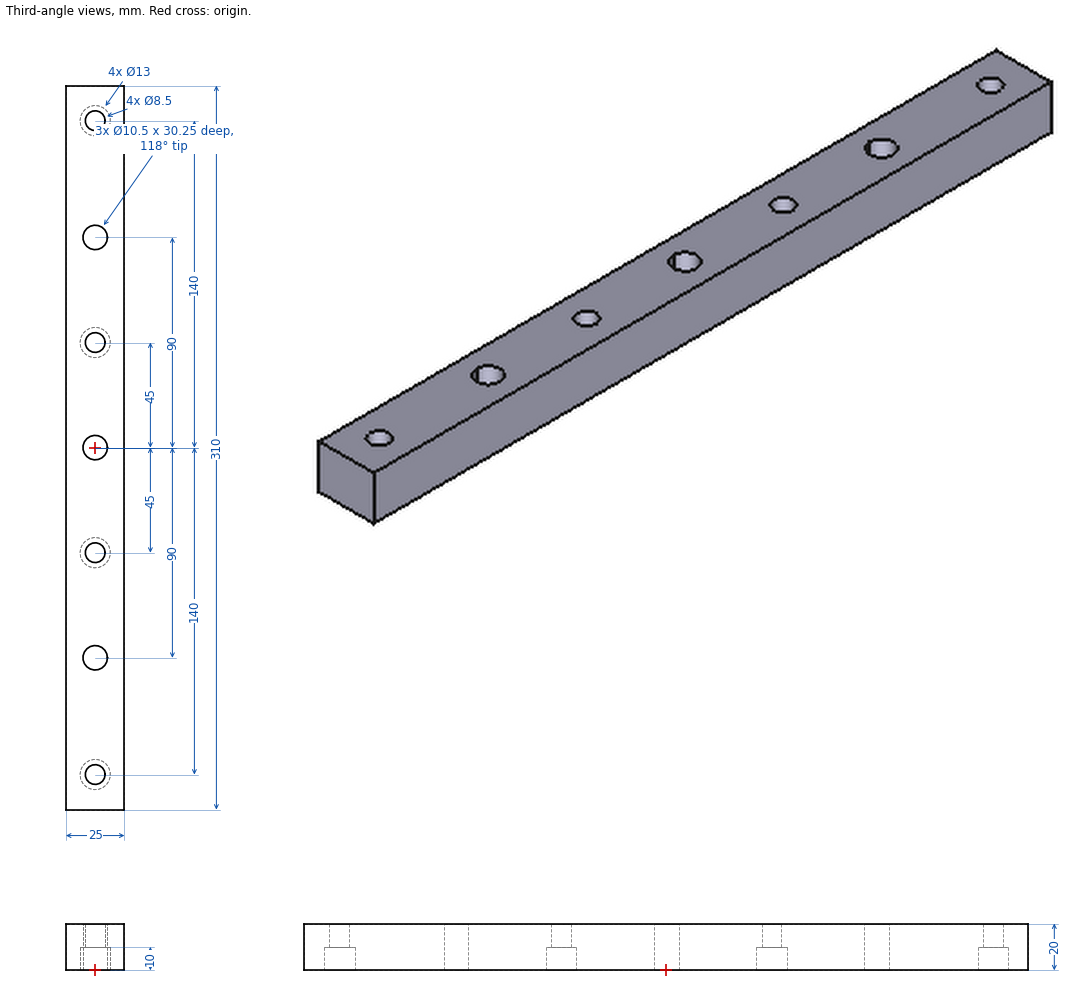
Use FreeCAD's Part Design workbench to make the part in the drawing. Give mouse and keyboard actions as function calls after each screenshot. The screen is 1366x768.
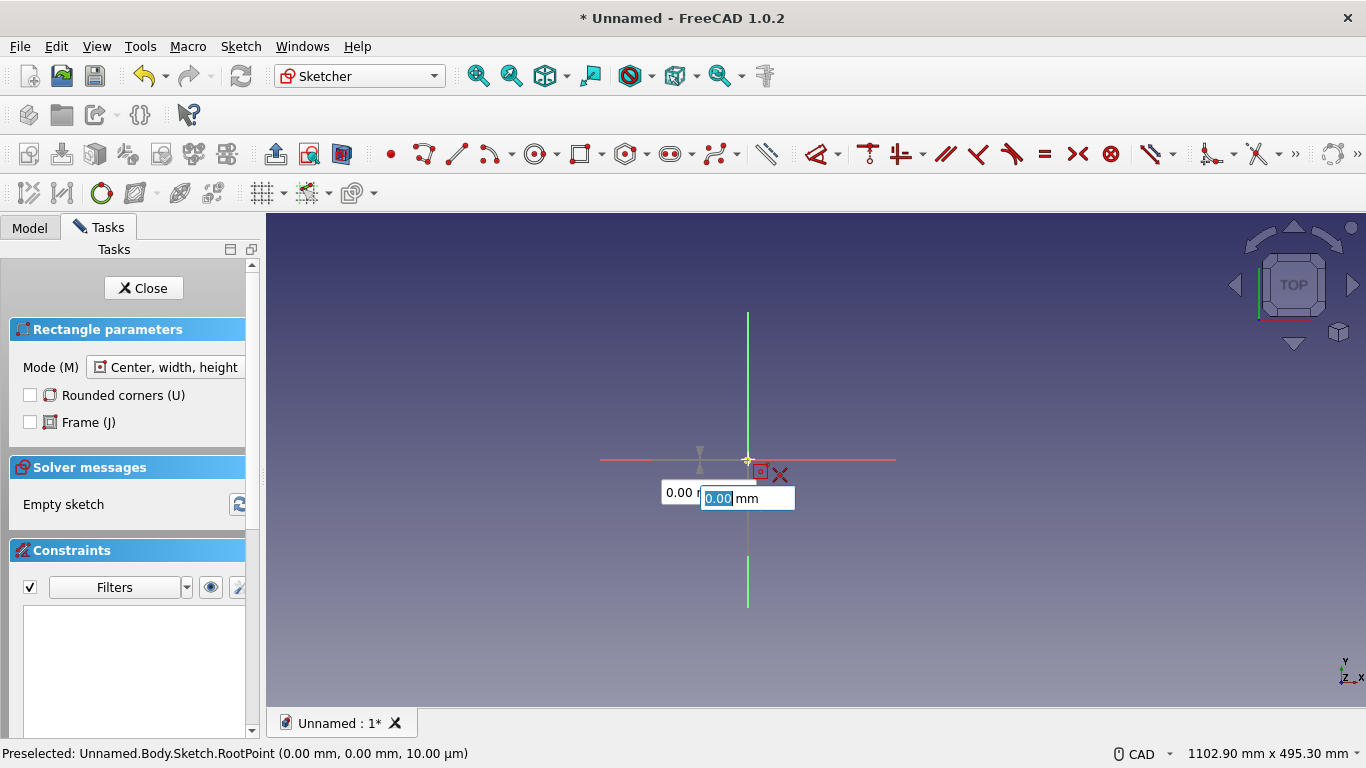
scroll(760, 305, up, 2)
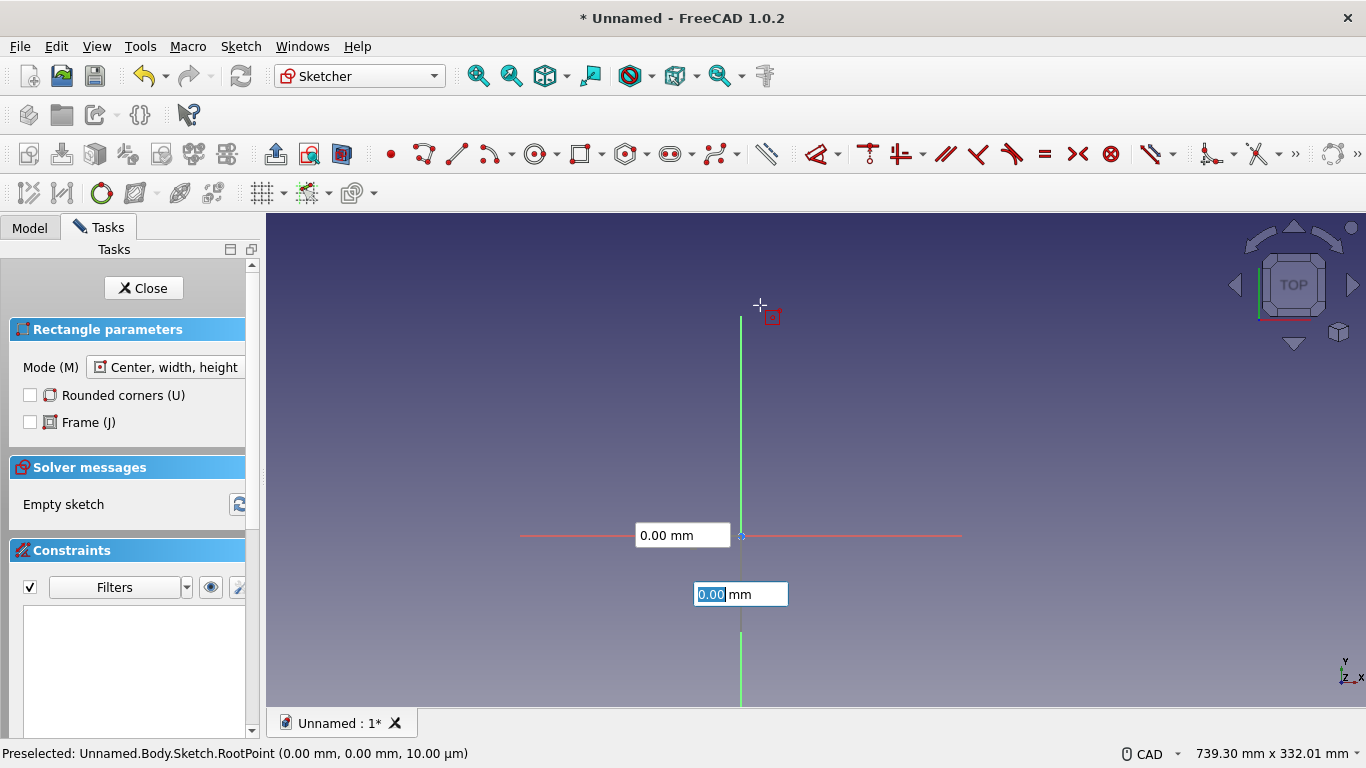
click(760, 306)
key(Escape)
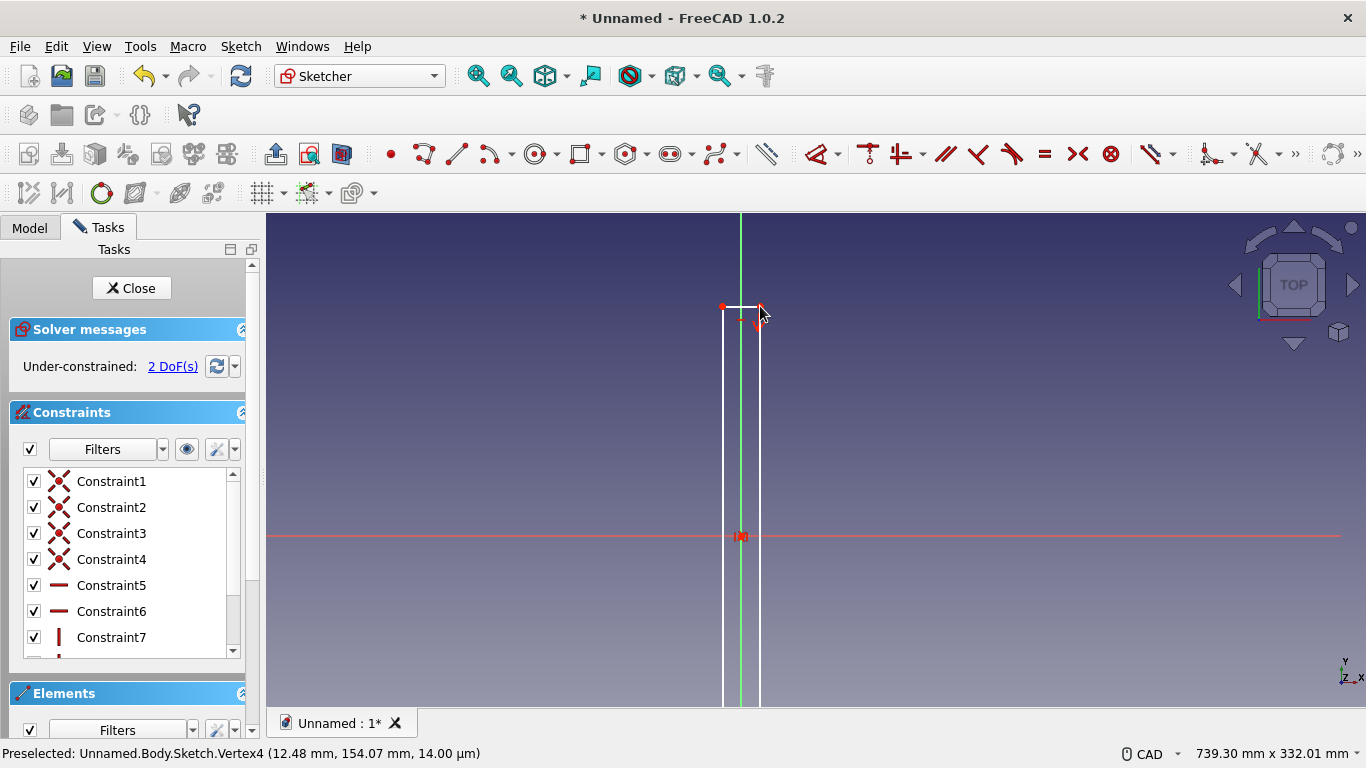
key(d)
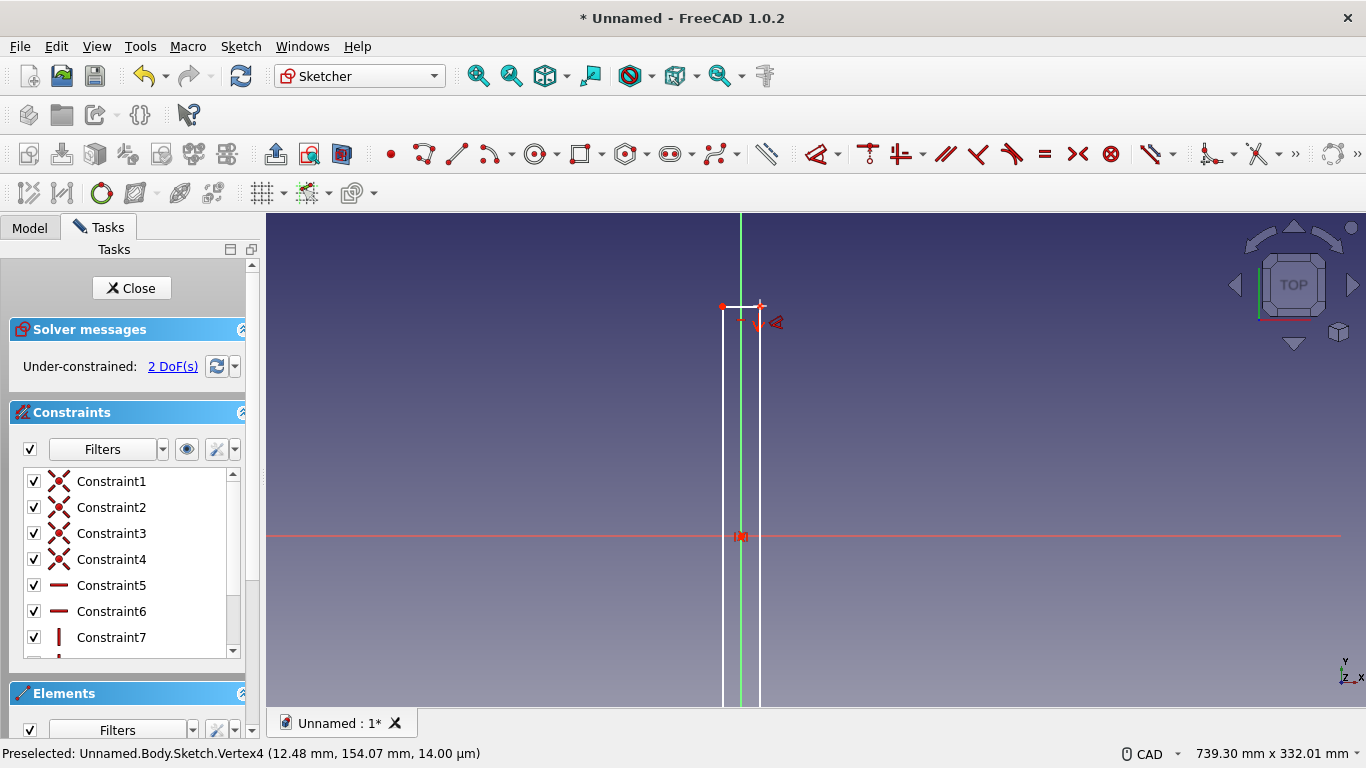
scroll(760, 305, down, 2)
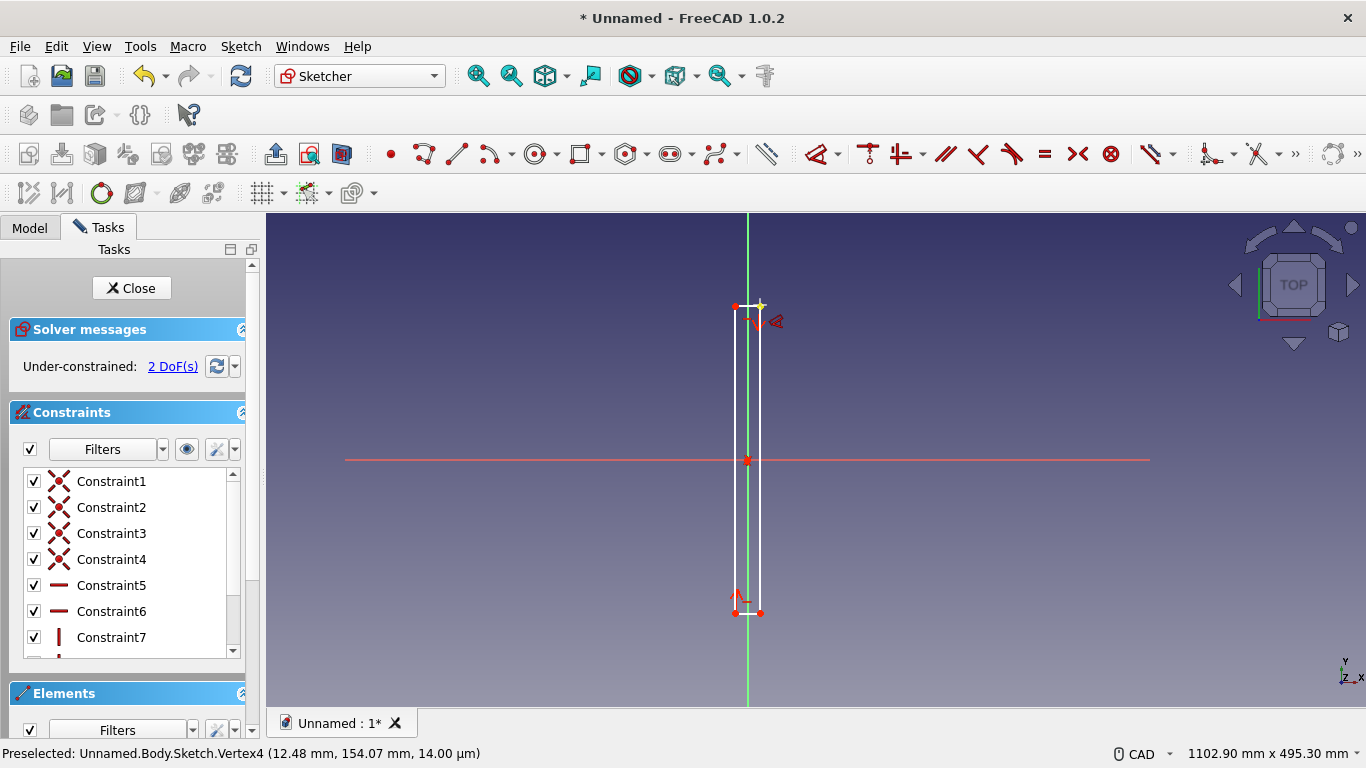
scroll(745, 614, up, 3)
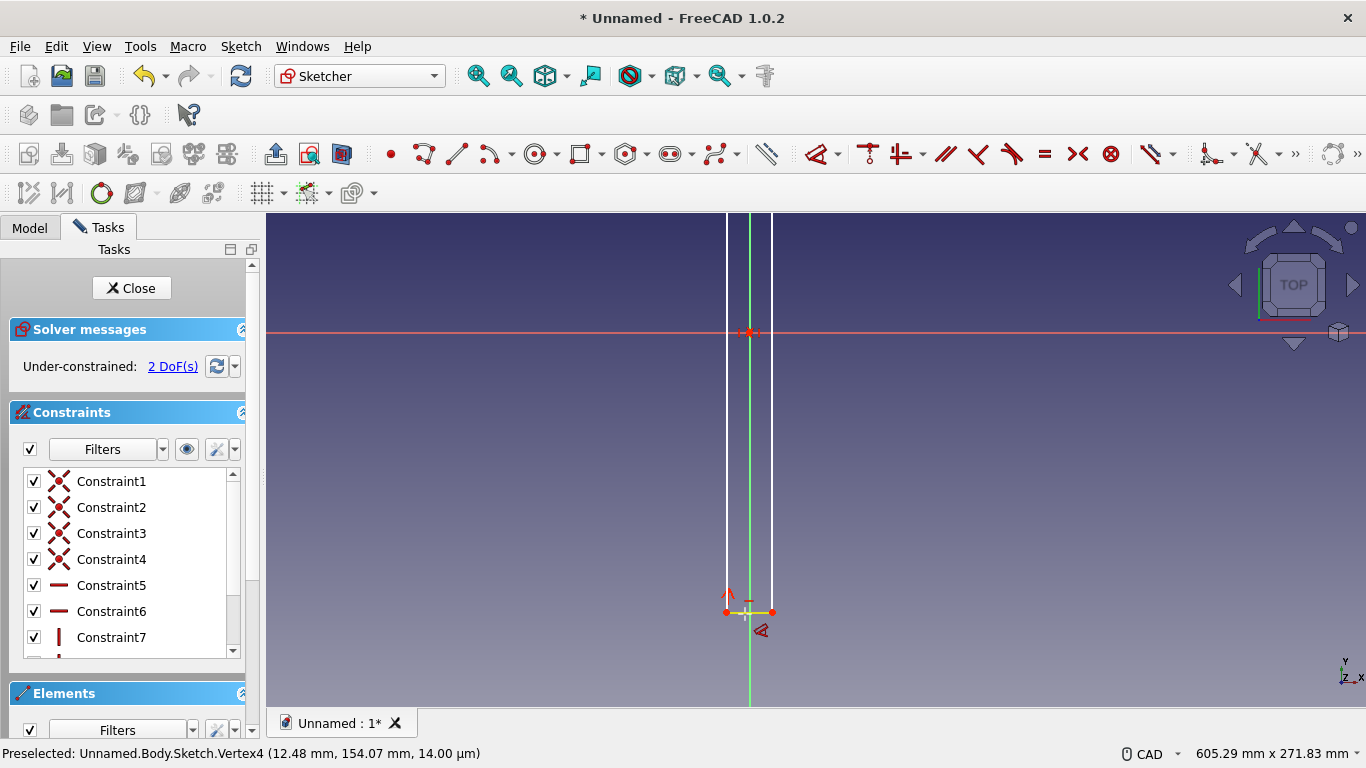
click(745, 613)
click(734, 647)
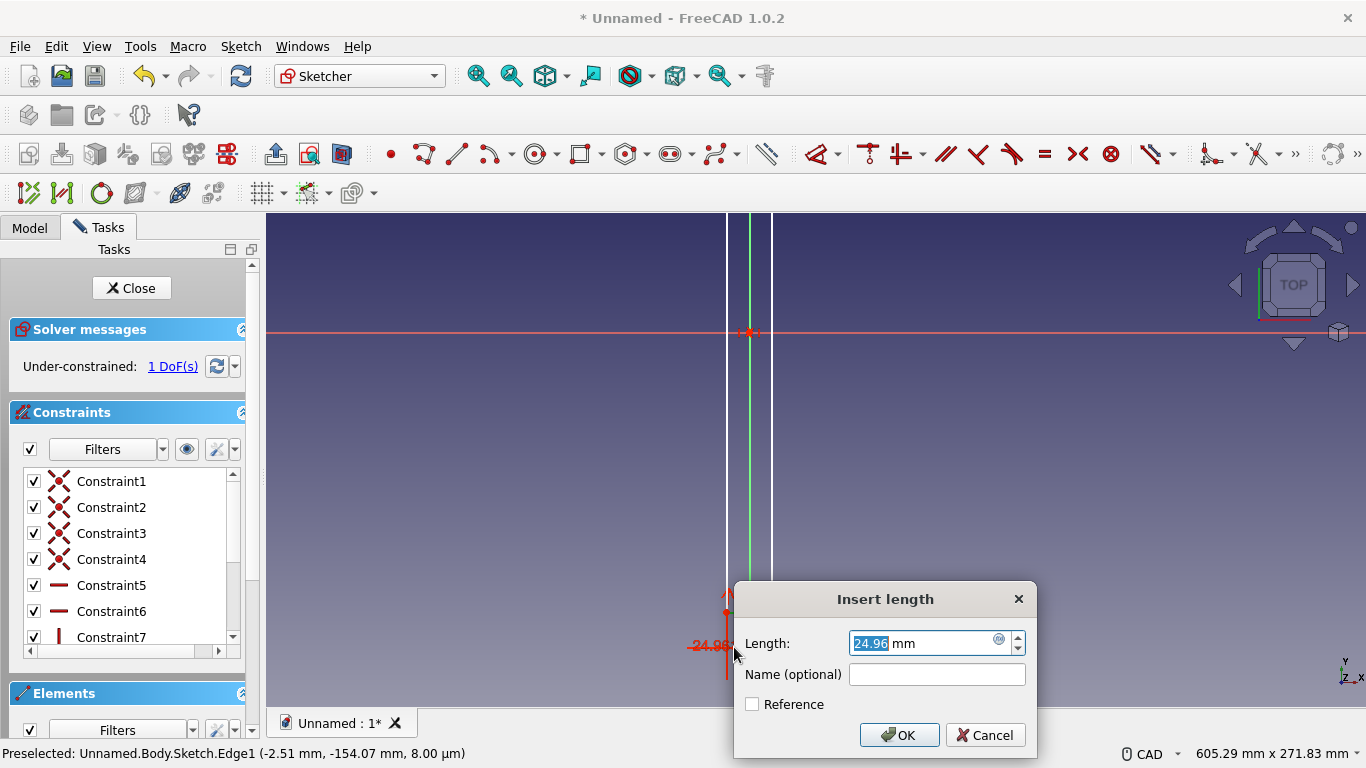
text(25)
key(Return)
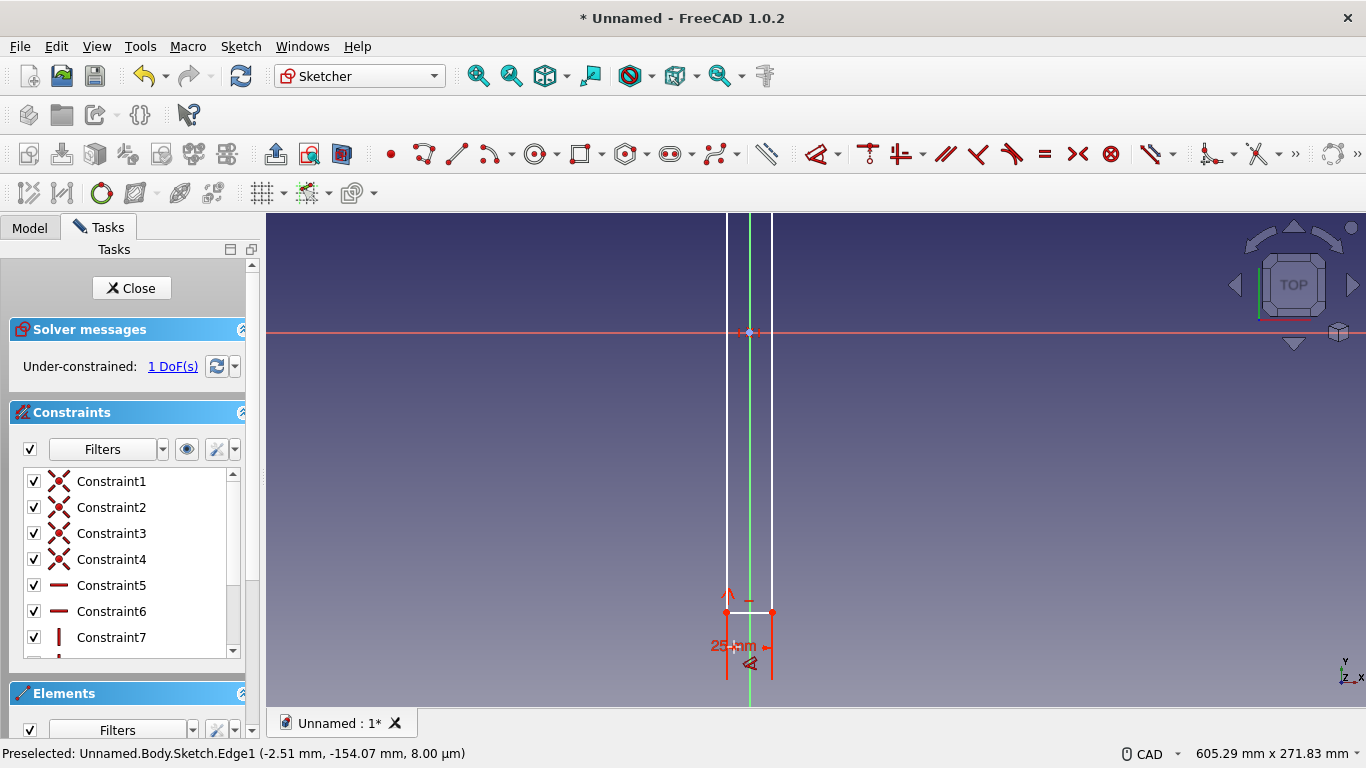
click(772, 445)
click(806, 427)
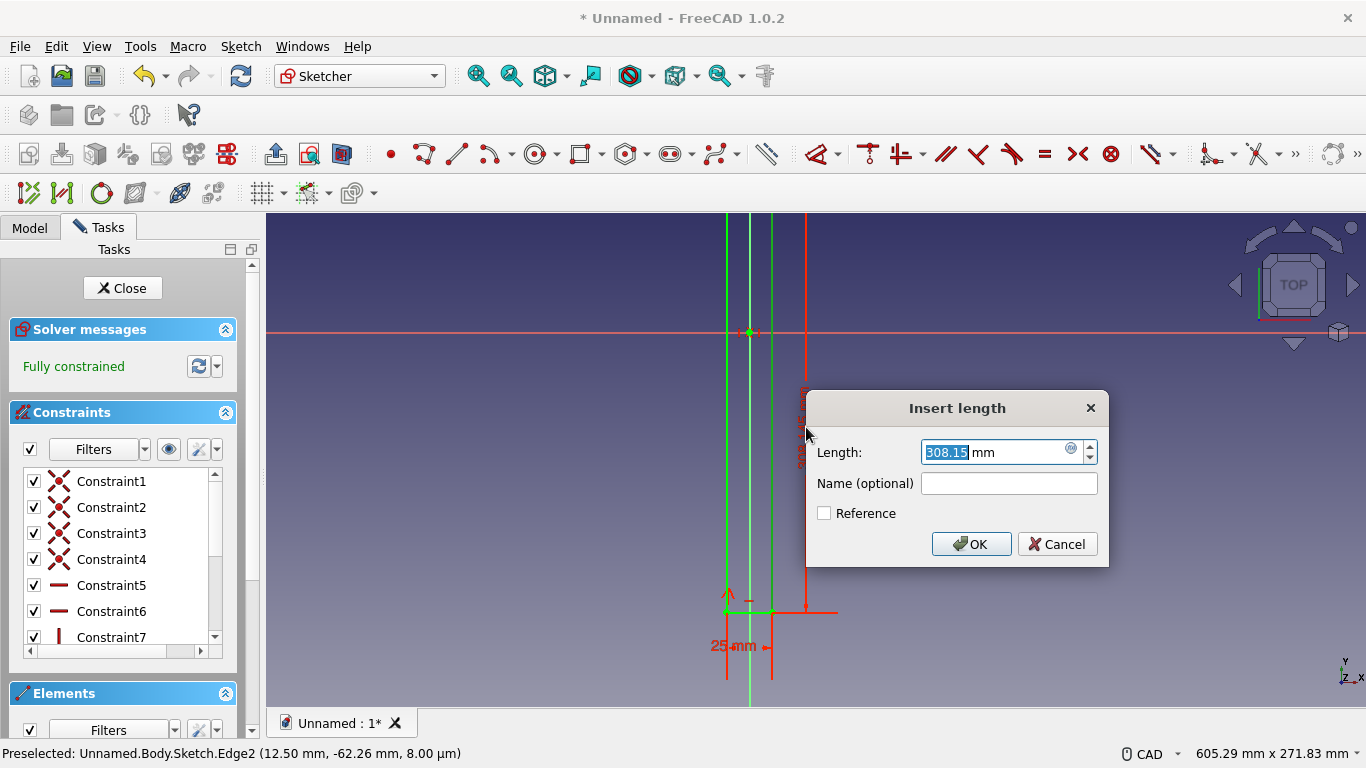
text(310)
key(Return)
key(Escape)